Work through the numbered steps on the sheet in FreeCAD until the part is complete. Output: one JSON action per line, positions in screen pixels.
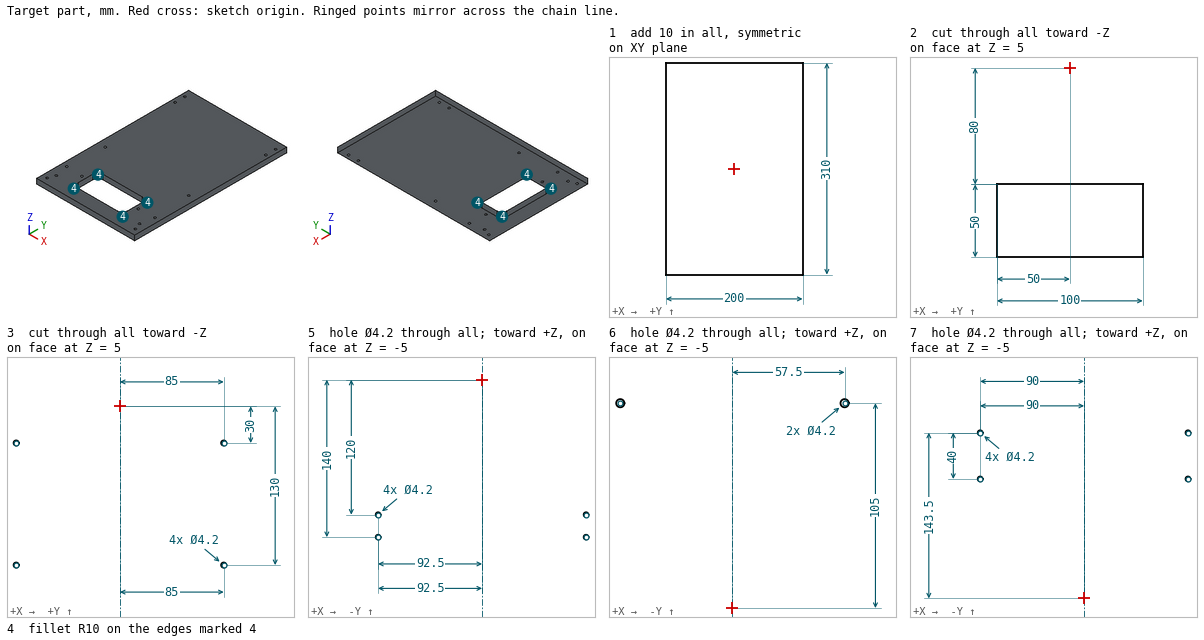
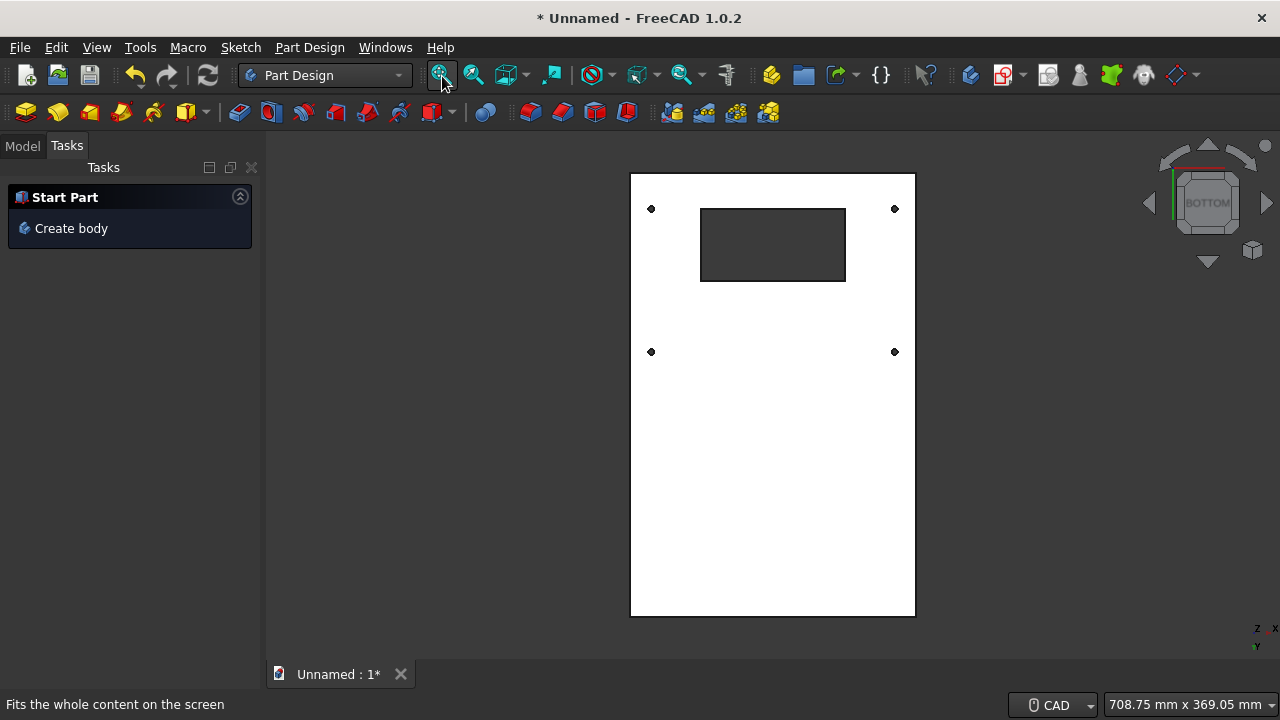
{"action": "scroll", "coordinate": [845, 280], "scroll_direction": "up", "scroll_amount": 6}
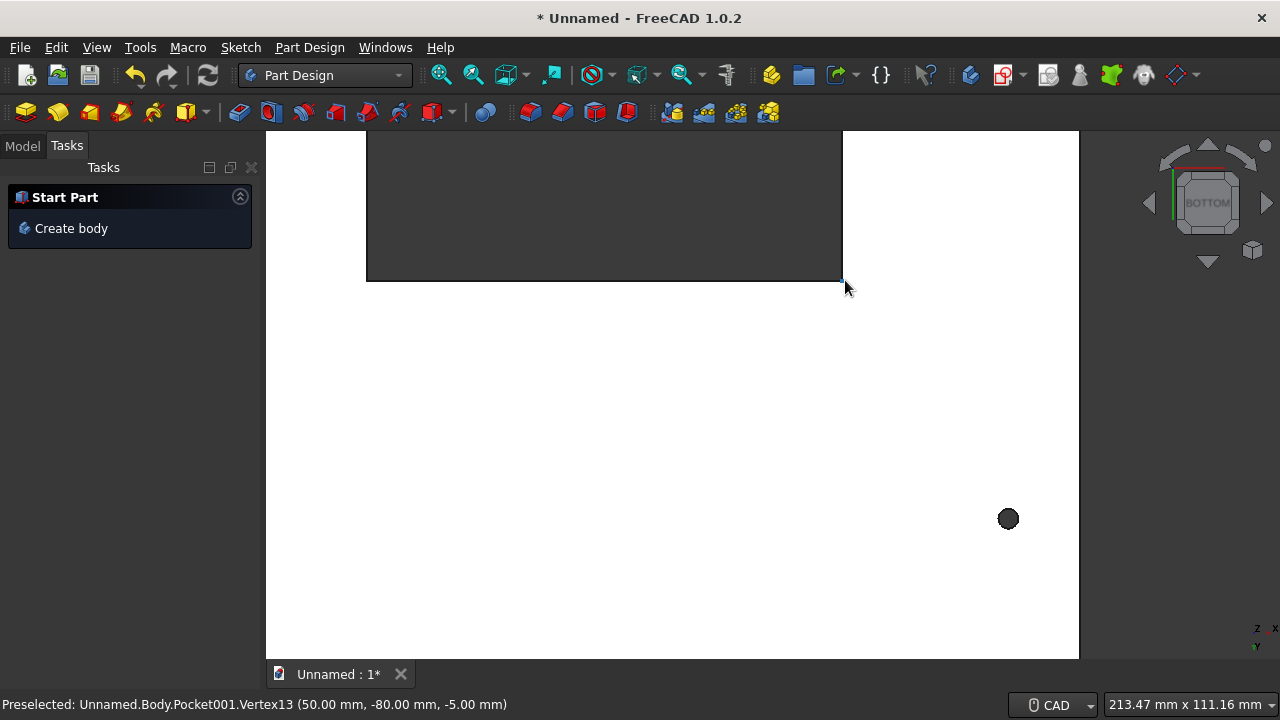
{"action": "left_click", "coordinate": [442, 76]}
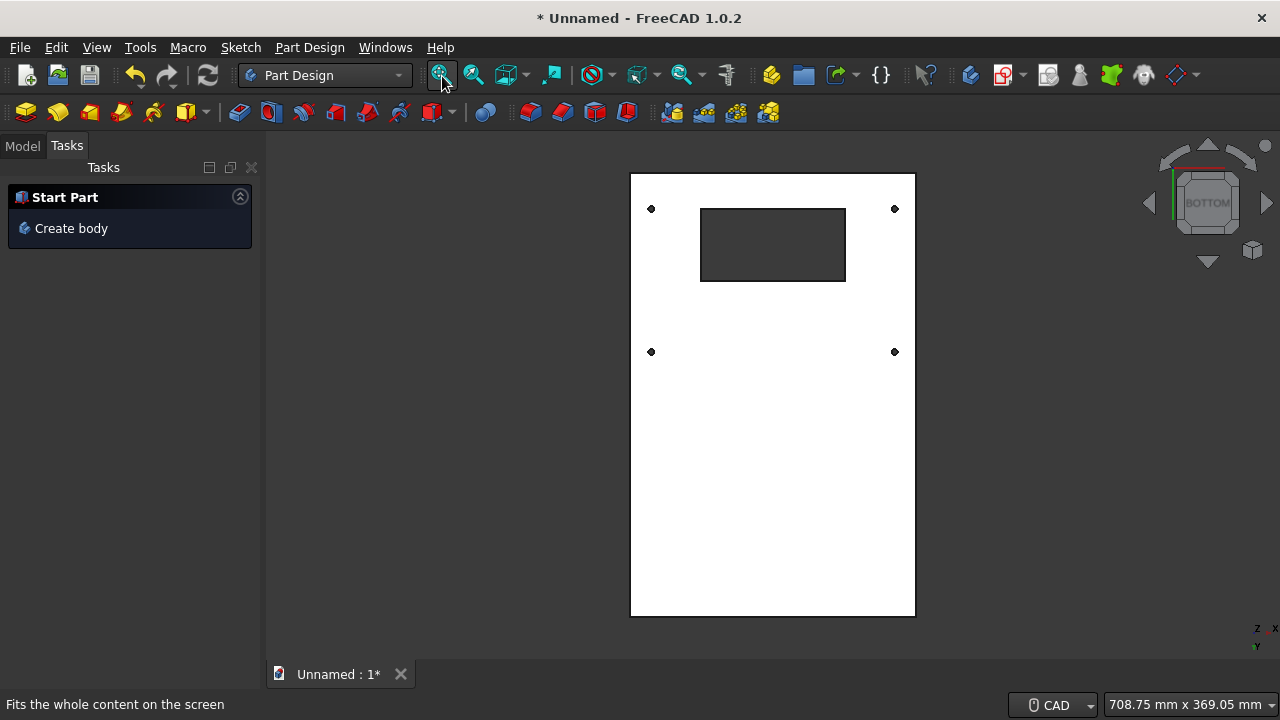
{"action": "key", "text": "4"}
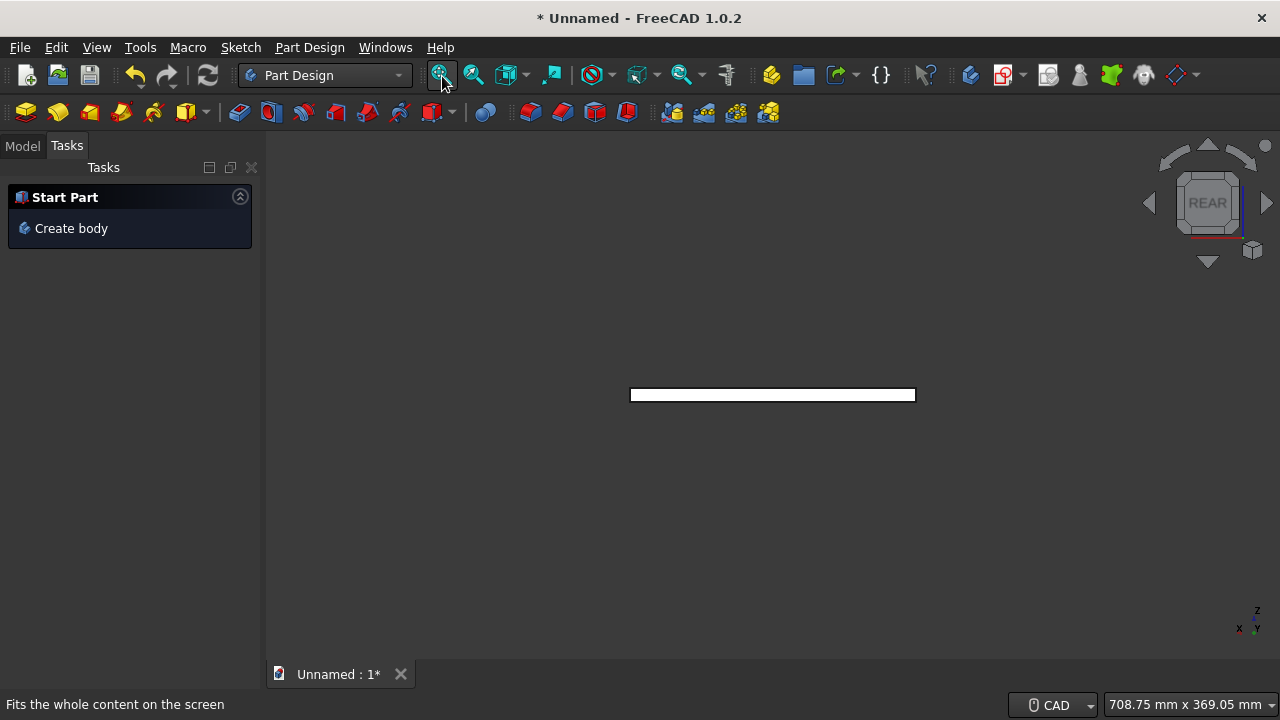
{"action": "left_click", "coordinate": [442, 76]}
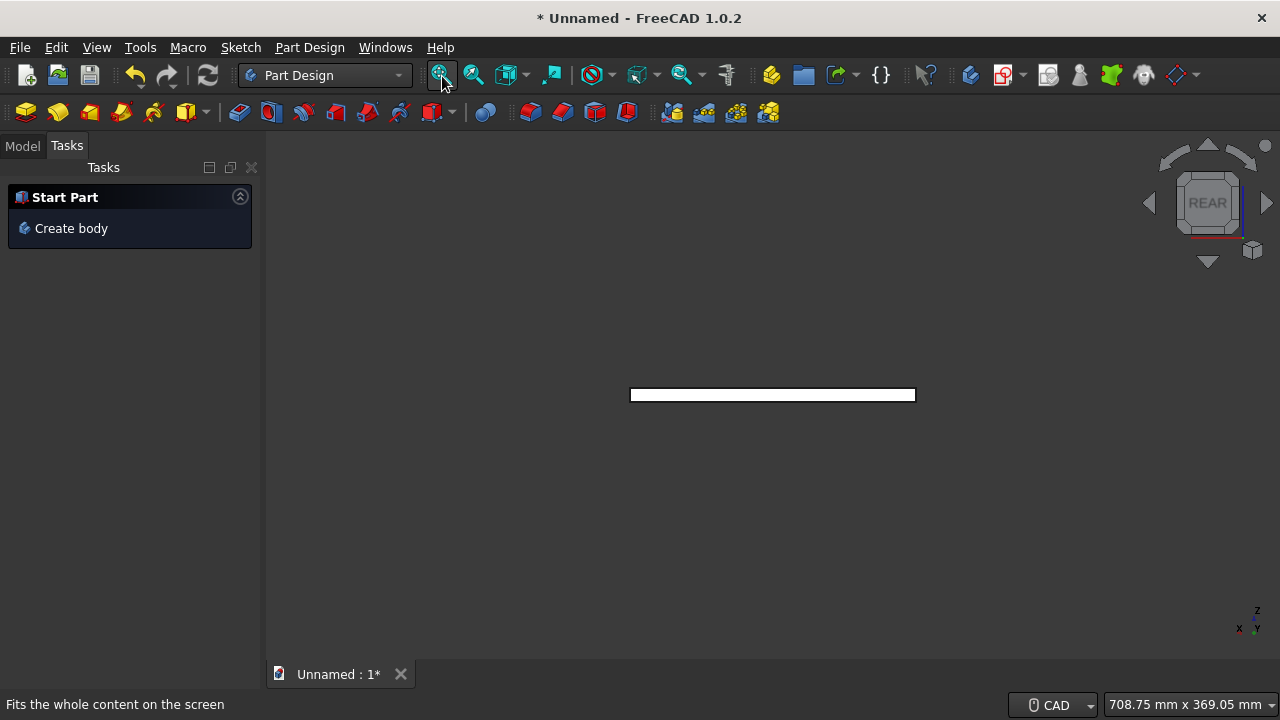
{"action": "scroll", "coordinate": [701, 394], "scroll_direction": "up", "scroll_amount": 6}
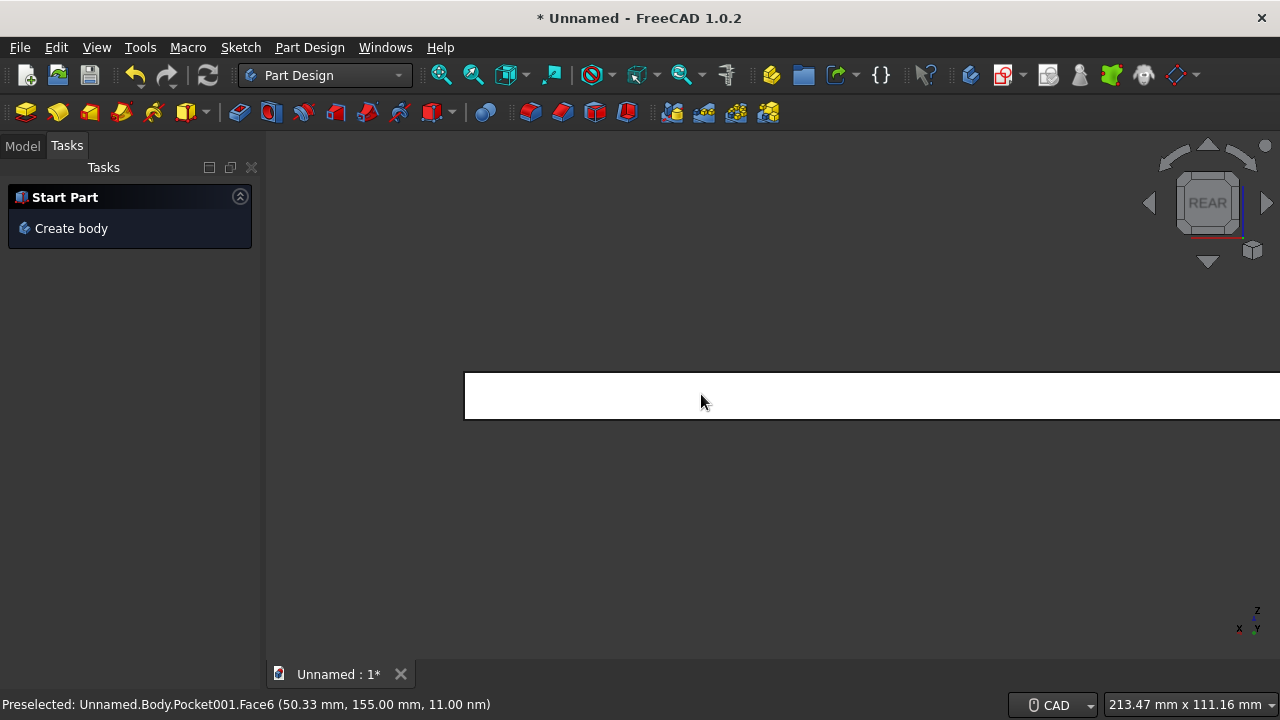
{"action": "left_click", "coordinate": [442, 76]}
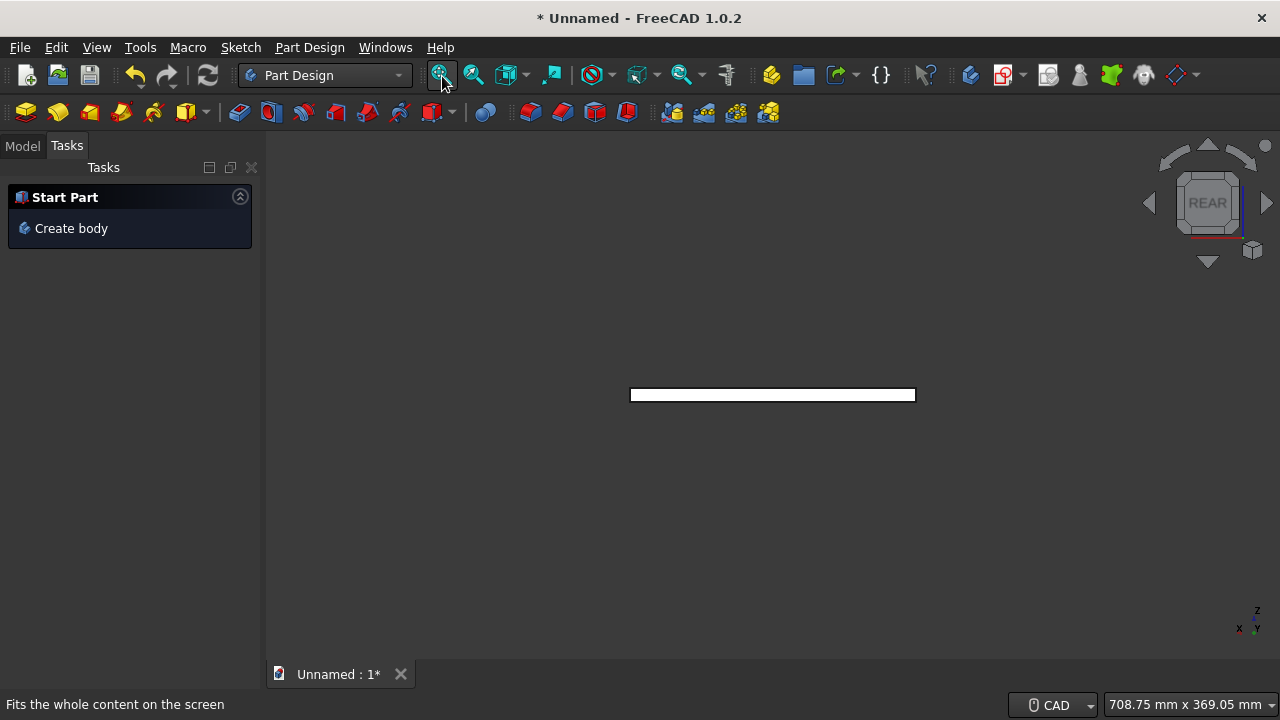
{"action": "key", "text": "6"}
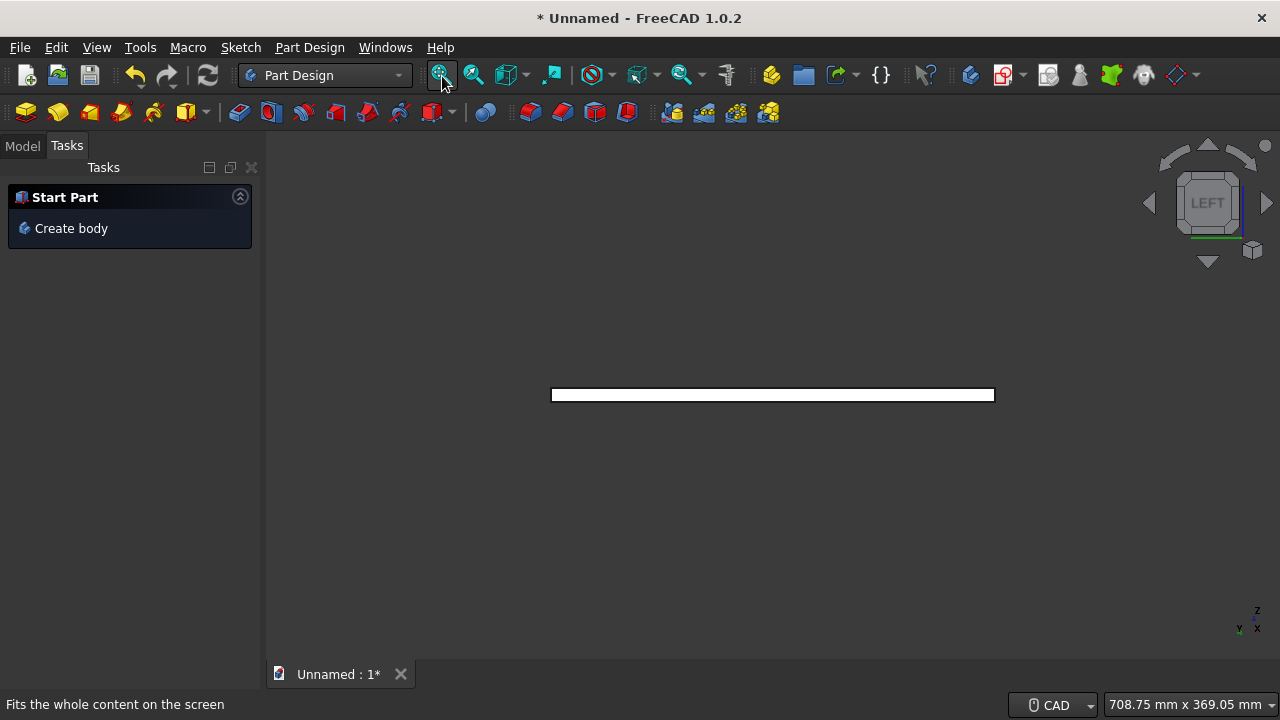
{"action": "left_click", "coordinate": [442, 76]}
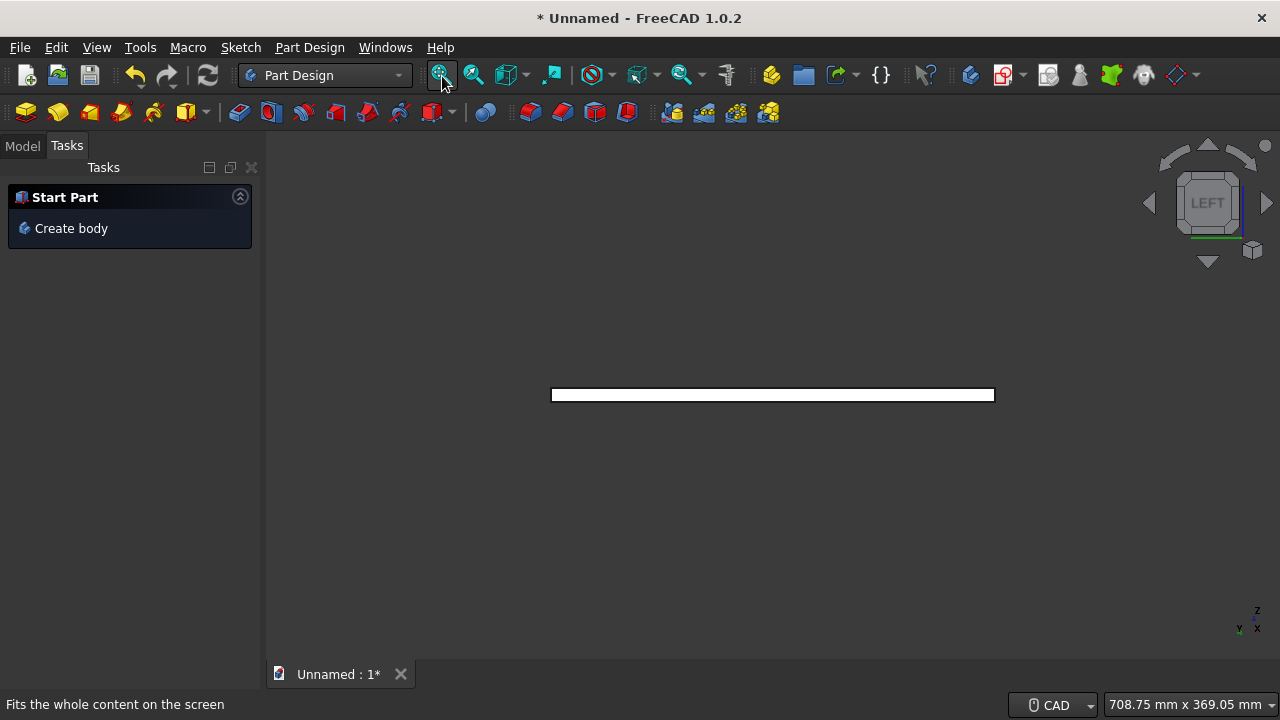
{"action": "scroll", "coordinate": [887, 394], "scroll_direction": "up", "scroll_amount": 6}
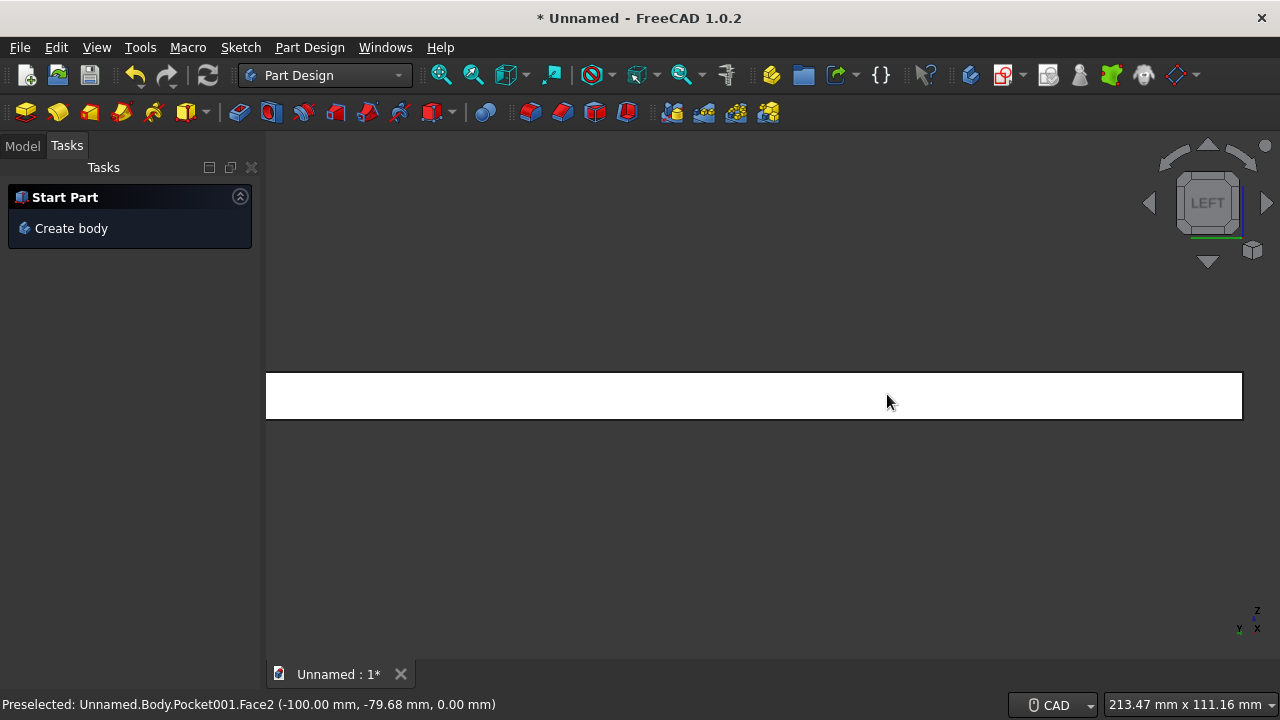
{"action": "left_click", "coordinate": [442, 76]}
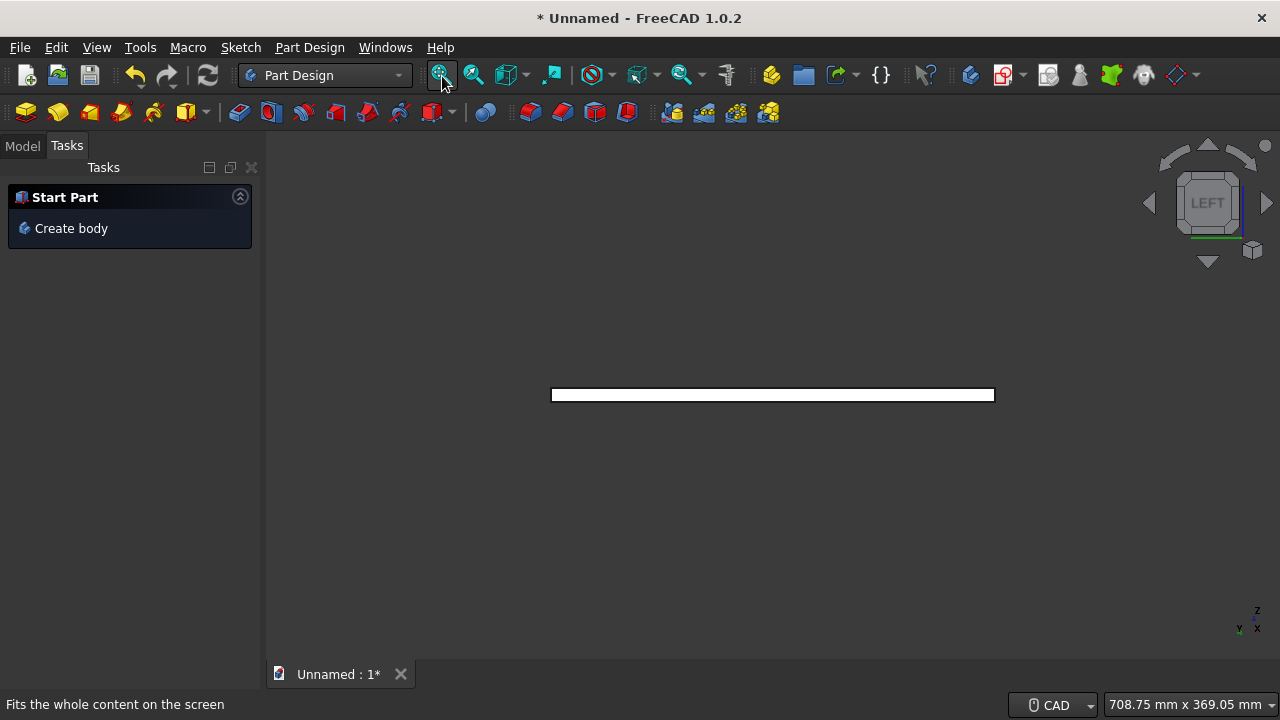
{"action": "key", "text": "v 3"}